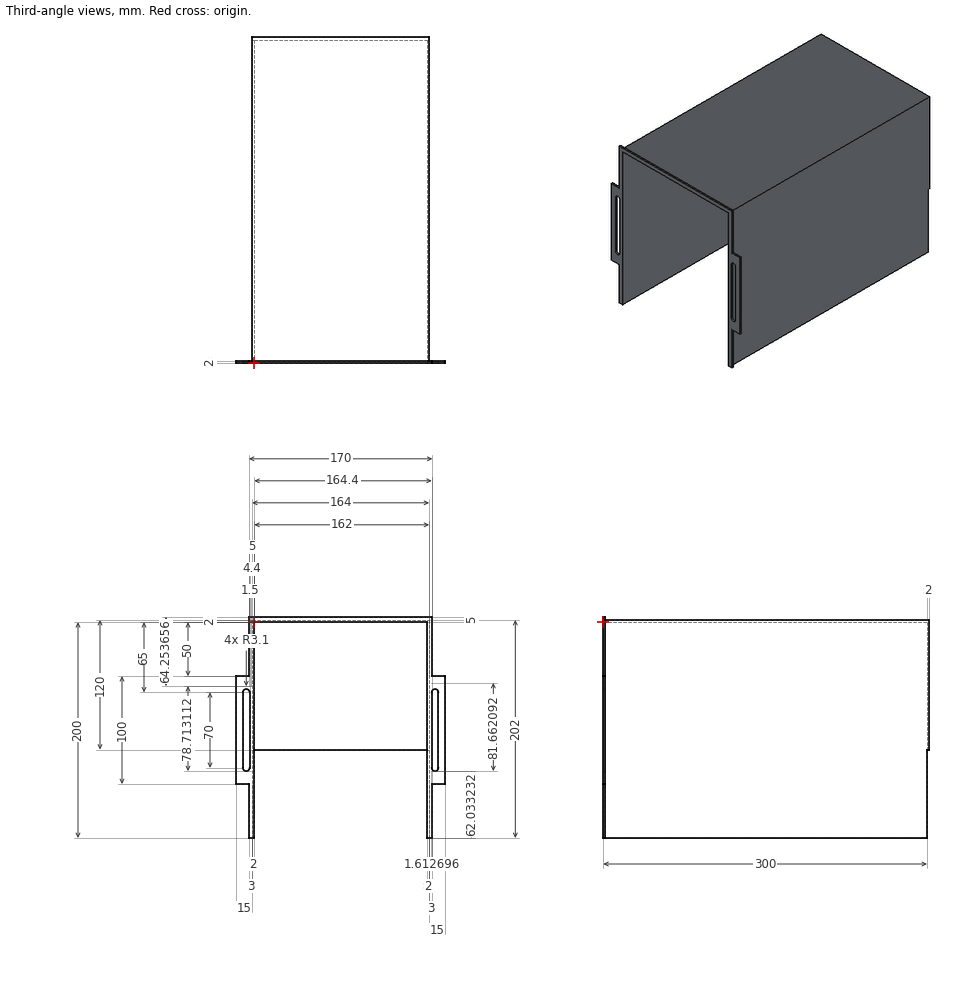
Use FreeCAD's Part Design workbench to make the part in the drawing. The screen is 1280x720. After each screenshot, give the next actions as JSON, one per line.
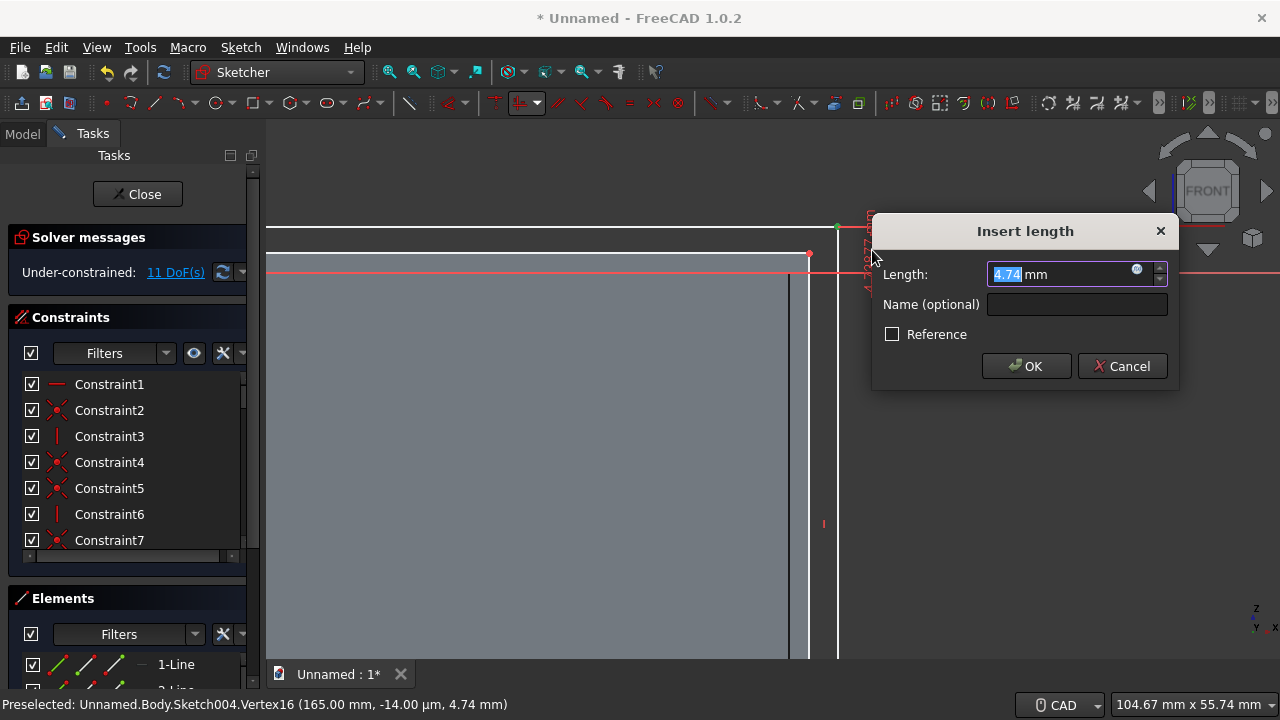
{"action": "type", "text": "5"}
{"action": "key", "text": "Return"}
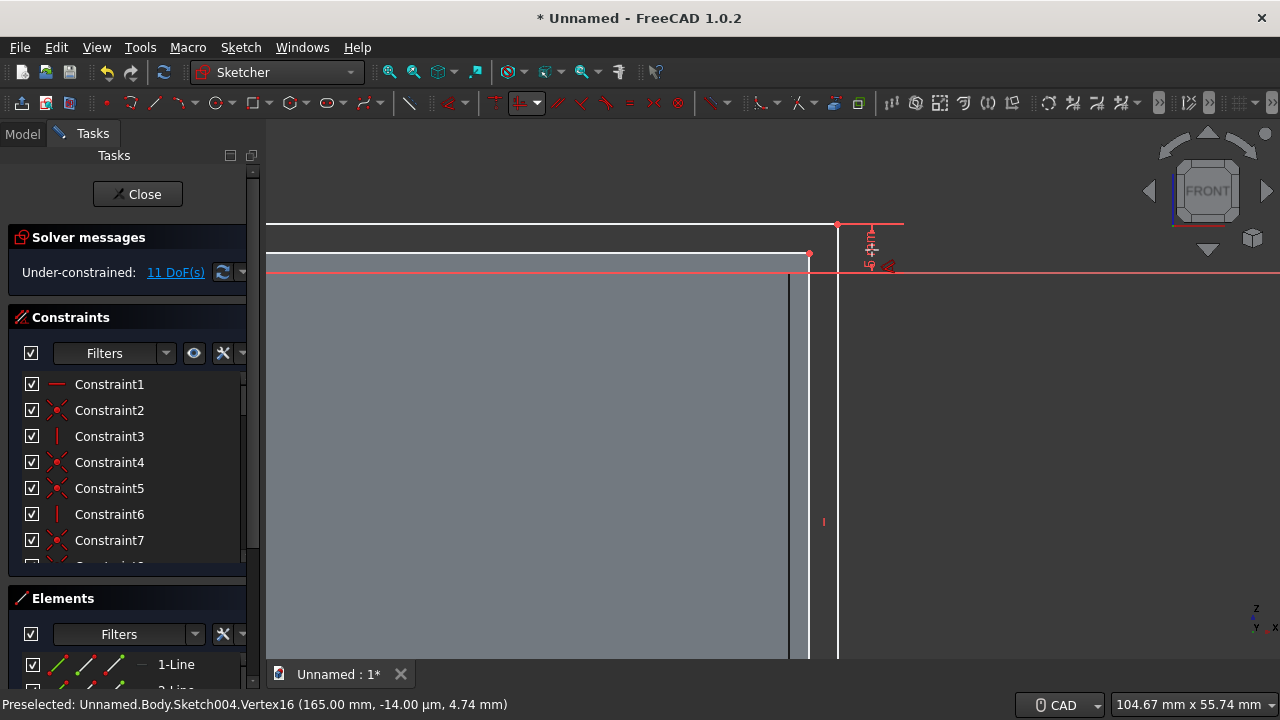
{"action": "scroll", "coordinate": [841, 225], "scroll_direction": "down", "scroll_amount": 9}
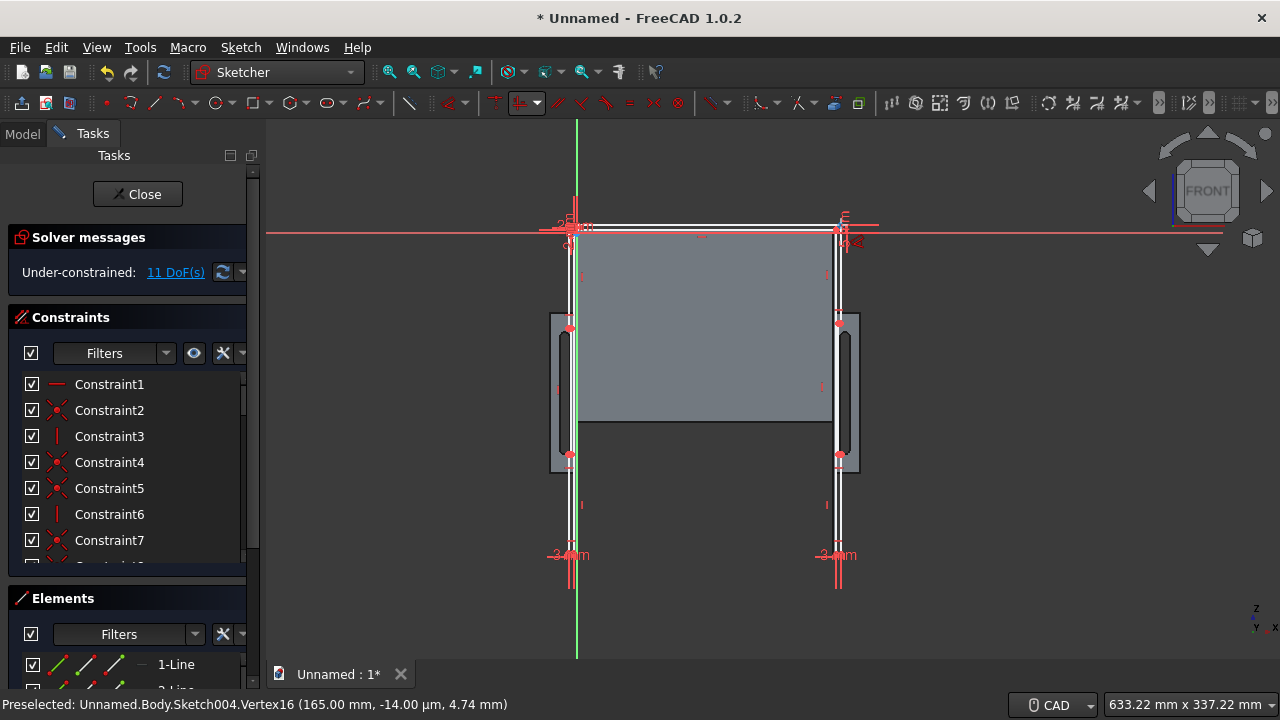
{"action": "scroll", "coordinate": [569, 225], "scroll_direction": "up", "scroll_amount": 9}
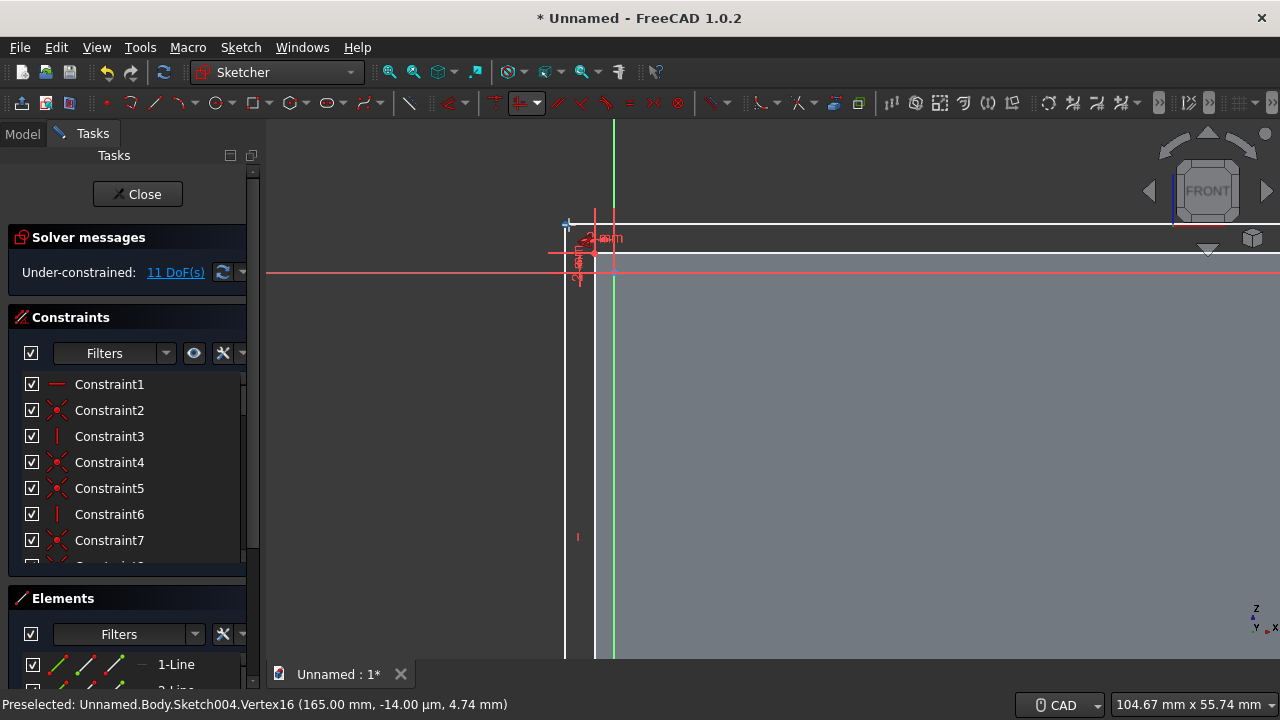
{"action": "left_click", "coordinate": [565, 224]}
{"action": "left_click", "coordinate": [590, 190]}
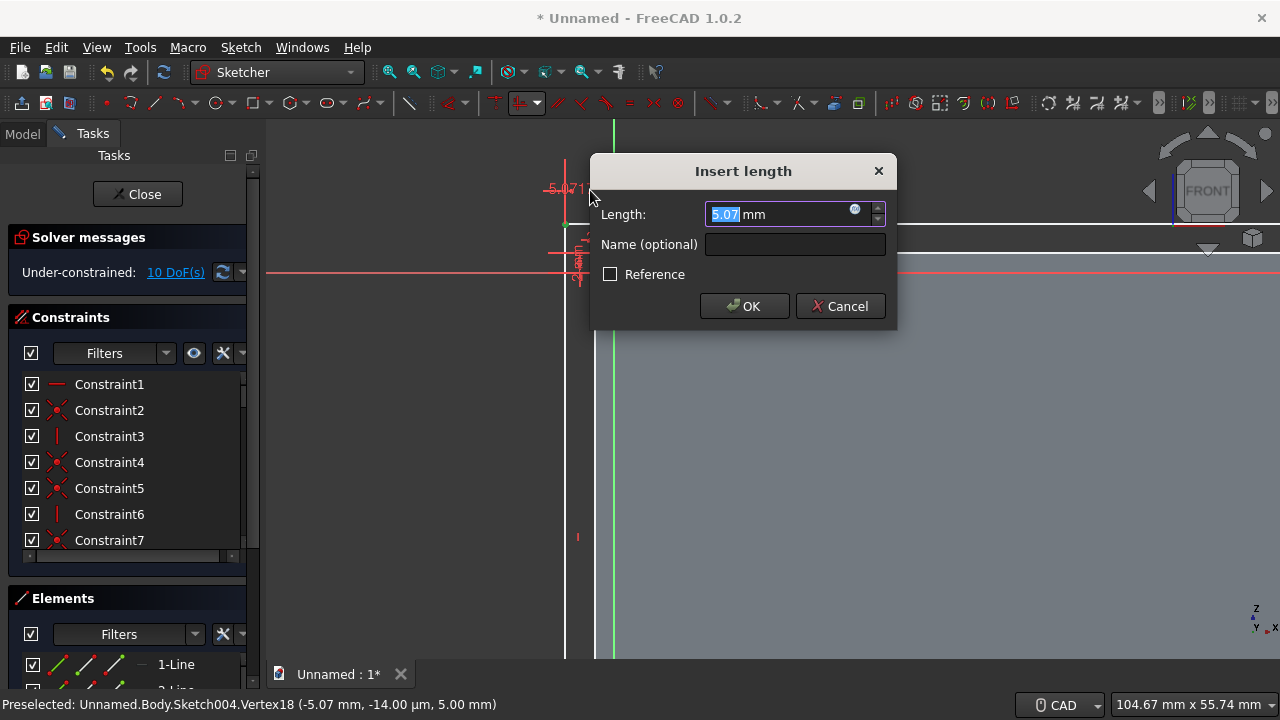
{"action": "type", "text": "5"}
{"action": "key", "text": "Return"}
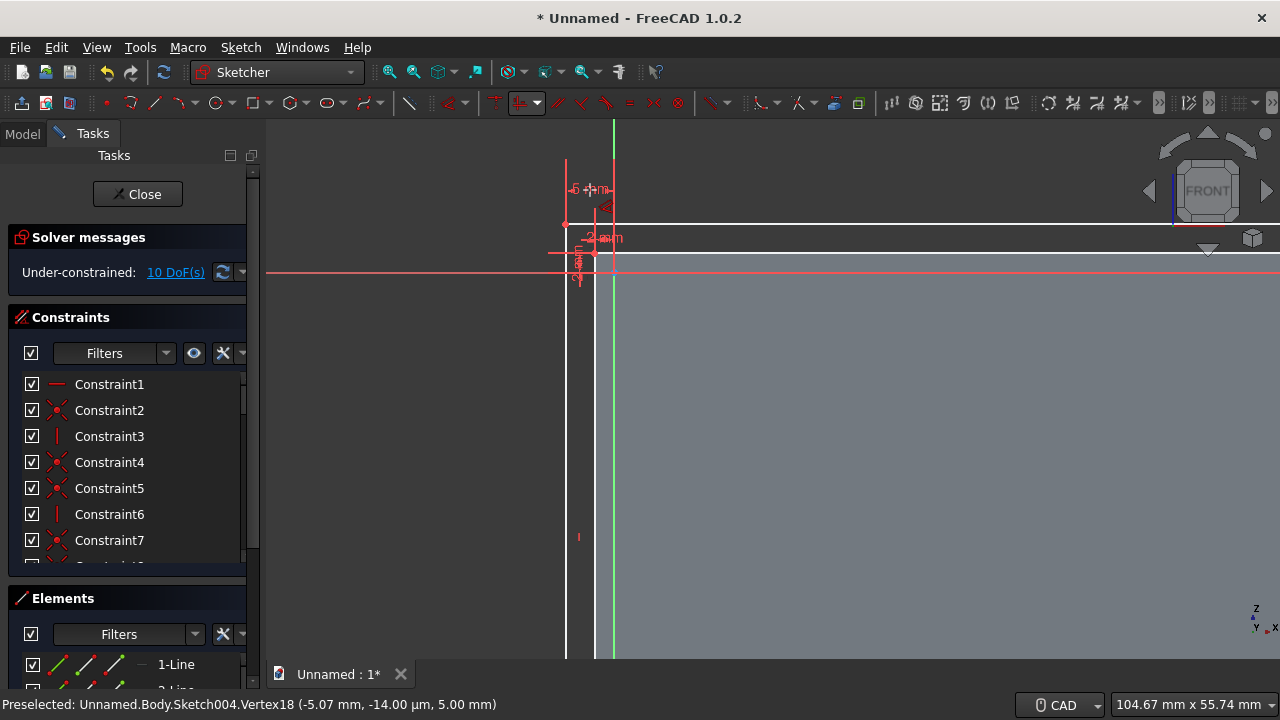
{"action": "left_click", "coordinate": [1072, 253]}
{"action": "left_click", "coordinate": [855, 287]}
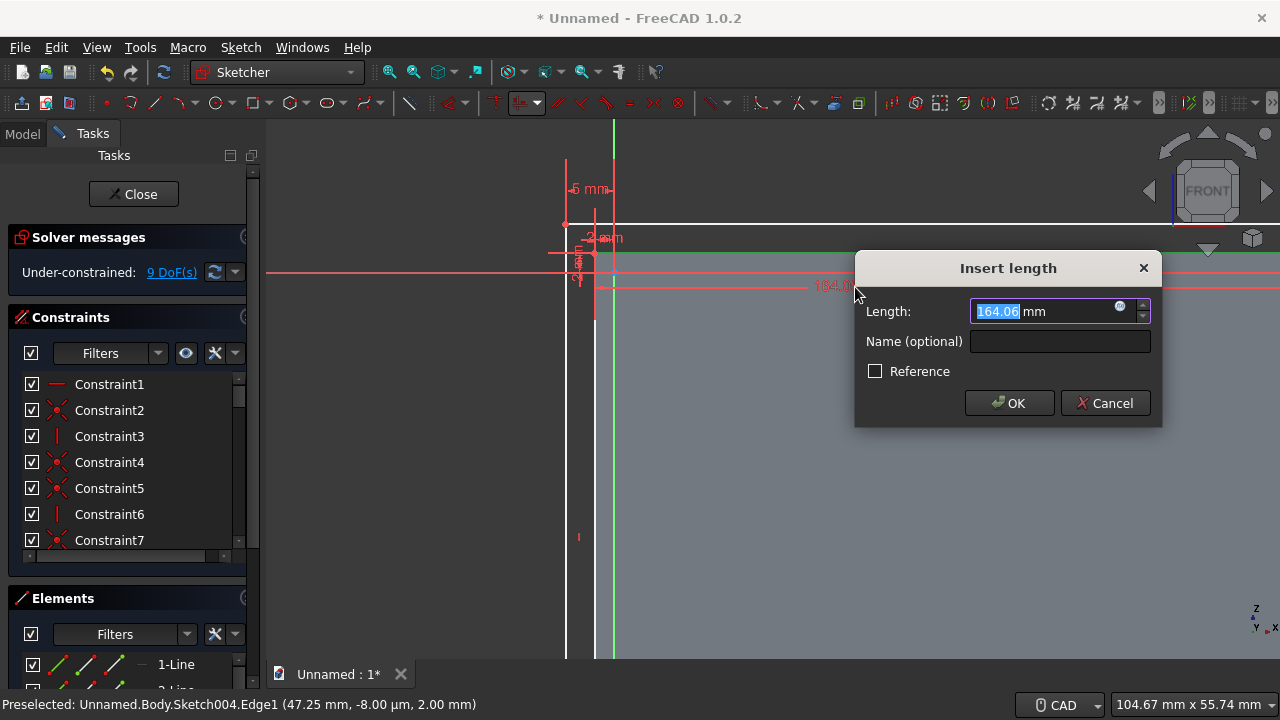
{"action": "type", "text": "164"}
{"action": "key", "text": "Return"}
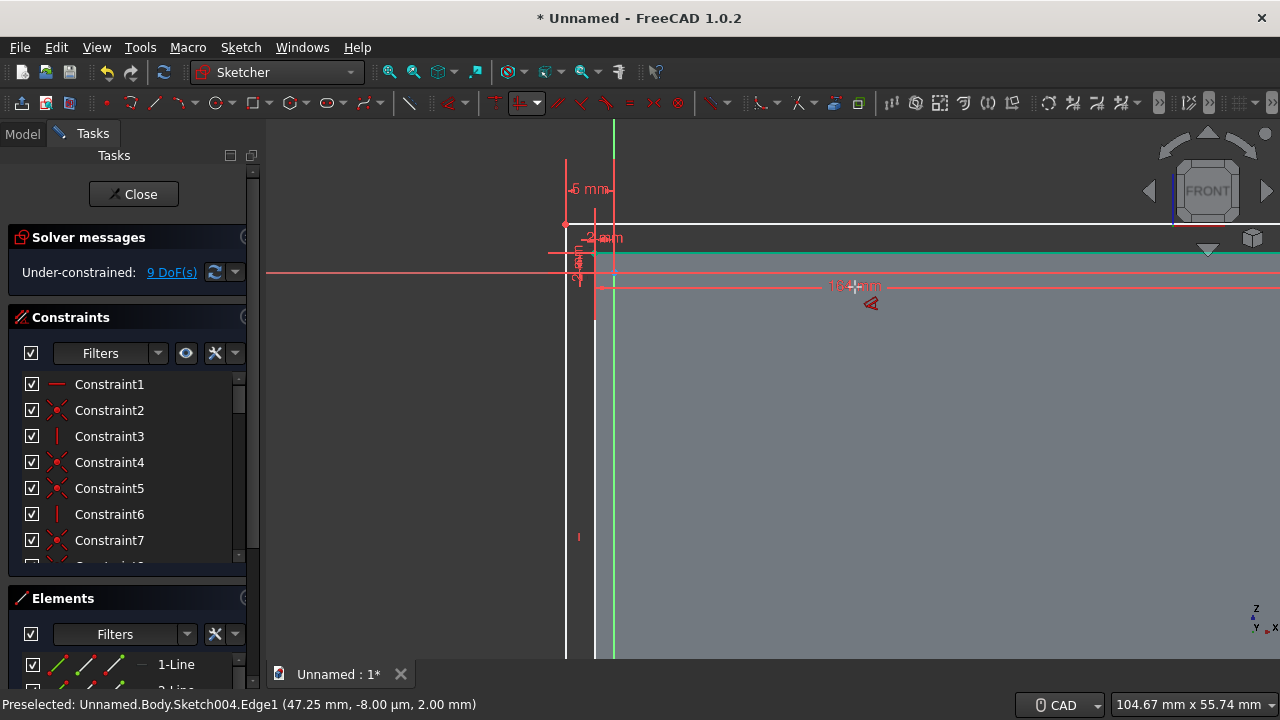
{"action": "scroll", "coordinate": [569, 225], "scroll_direction": "down", "scroll_amount": 9}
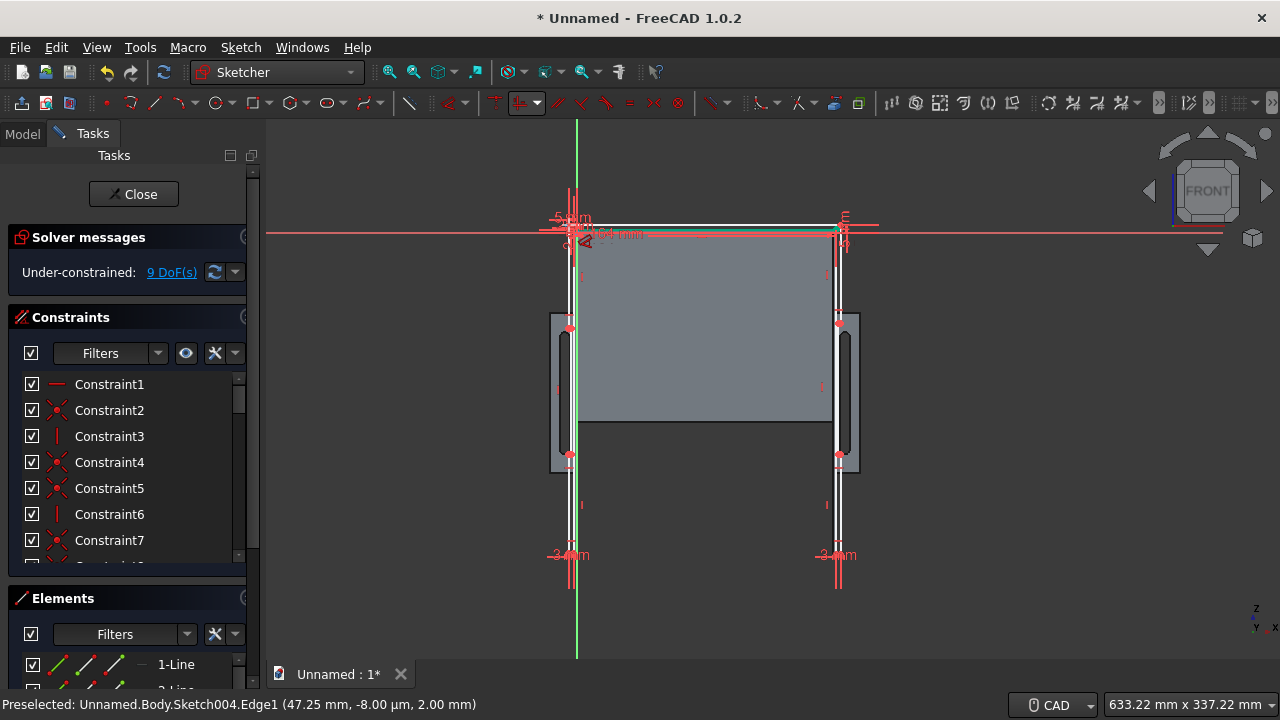
{"action": "scroll", "coordinate": [836, 327], "scroll_direction": "up", "scroll_amount": 10}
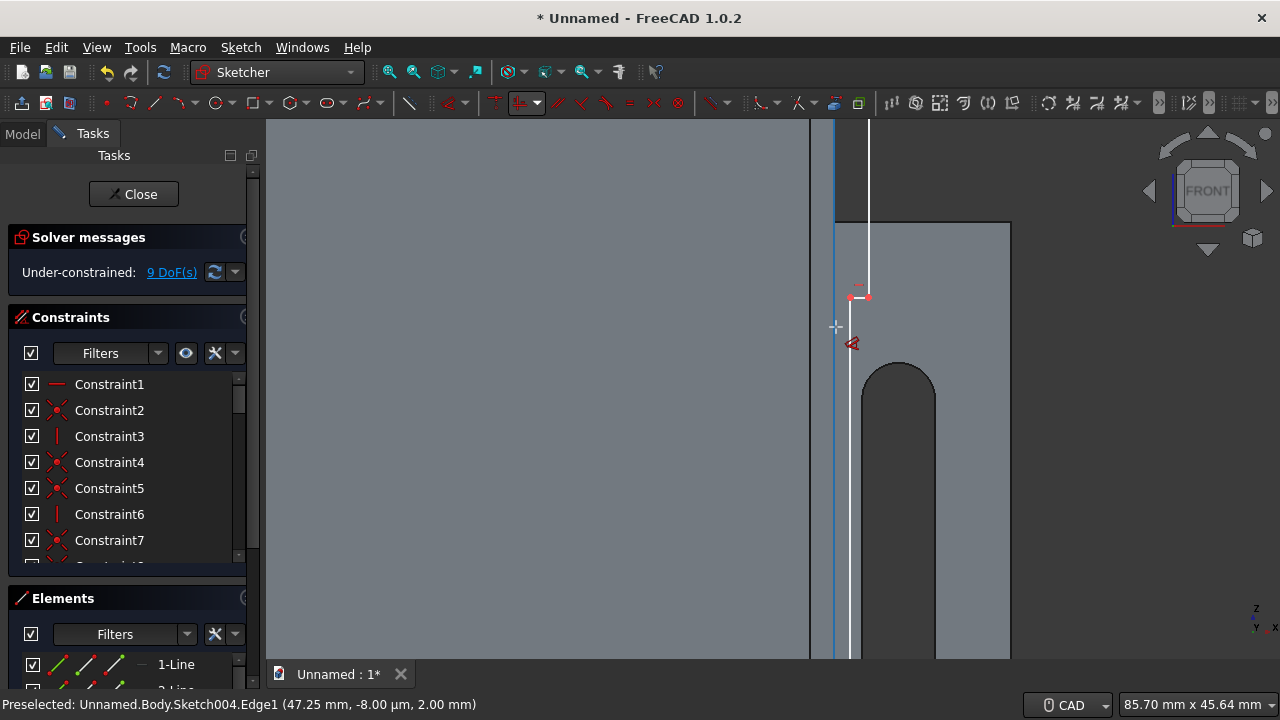
{"action": "left_click", "coordinate": [834, 325]}
{"action": "left_click", "coordinate": [868, 389]}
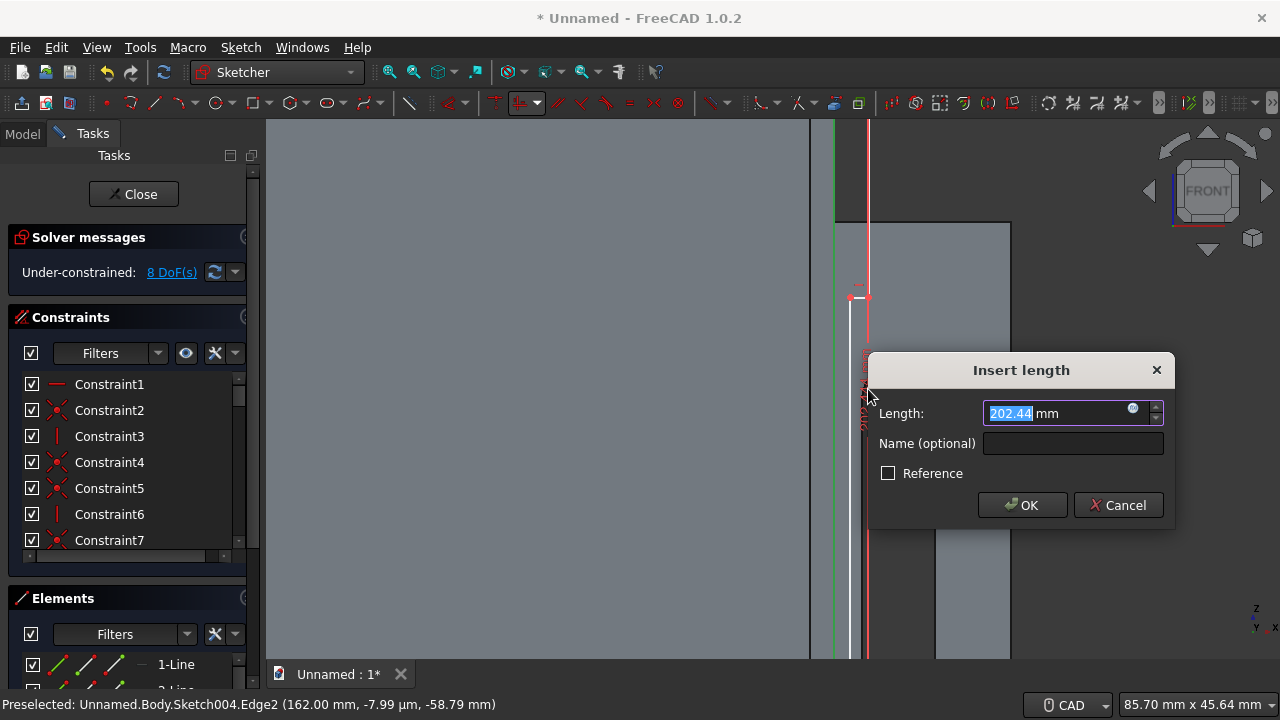
{"action": "type", "text": "202"}
{"action": "key", "text": "Return"}